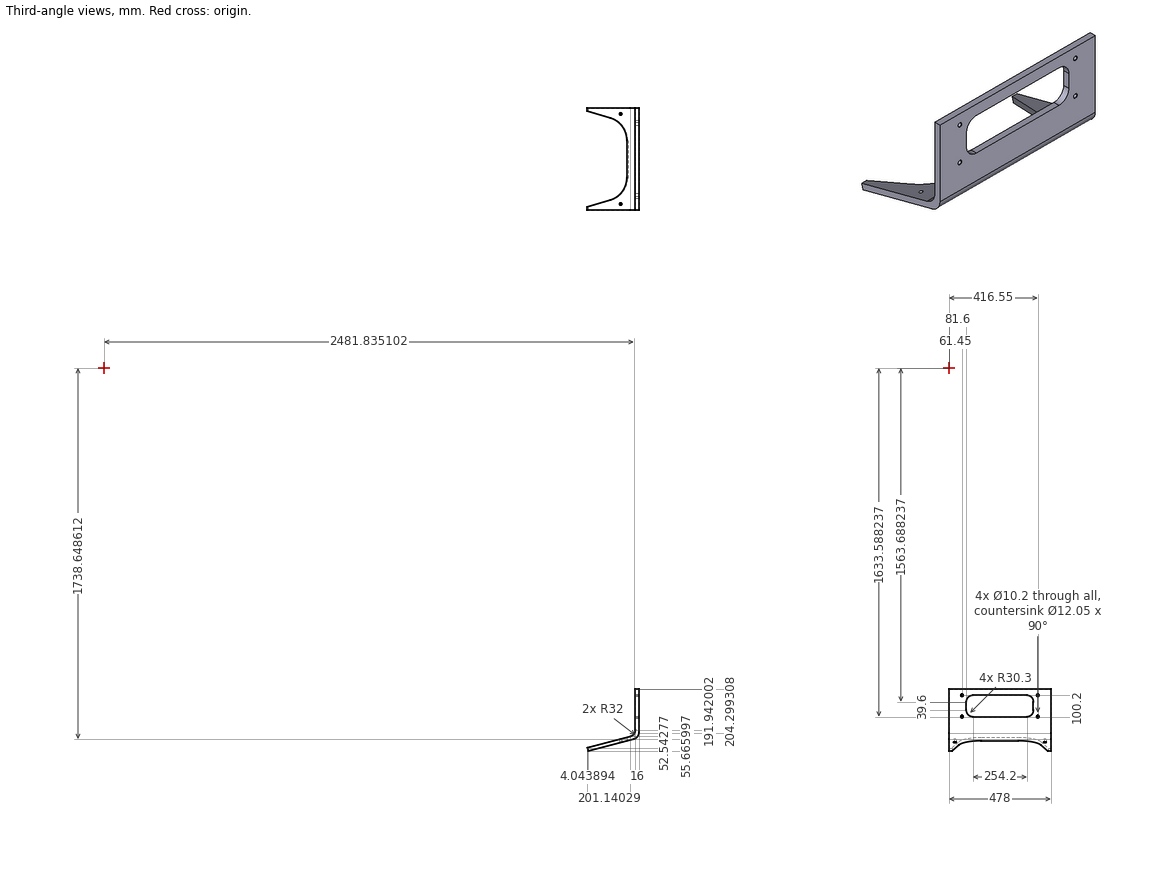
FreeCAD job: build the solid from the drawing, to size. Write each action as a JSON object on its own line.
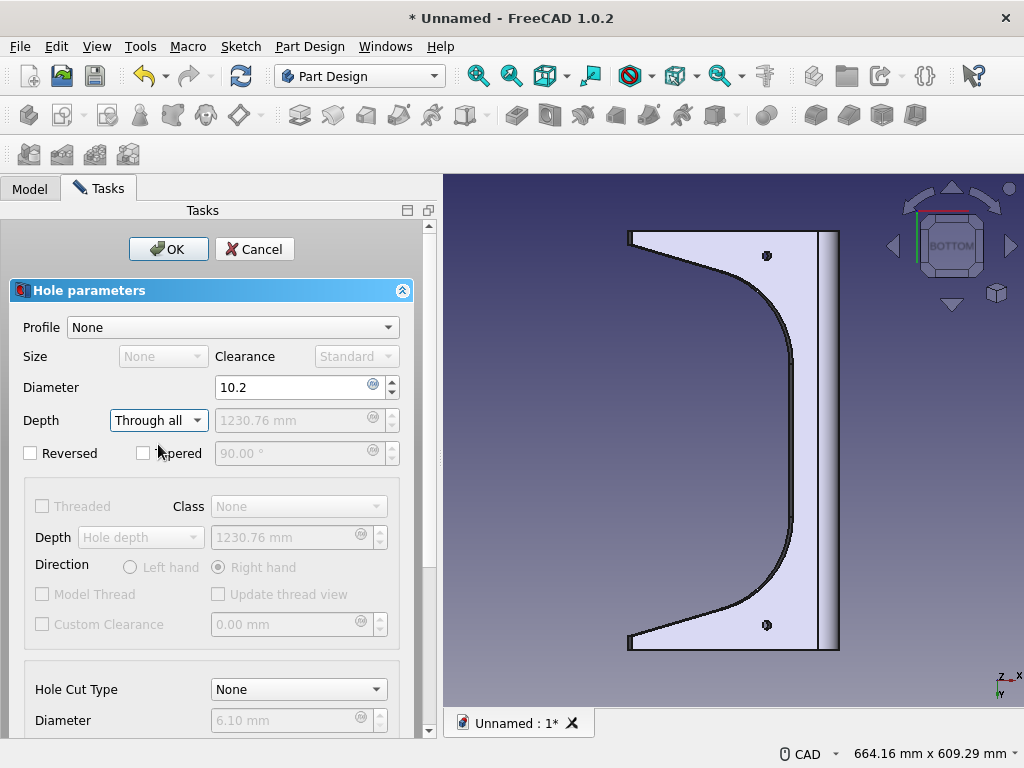
{"action": "left_click", "coordinate": [300, 690]}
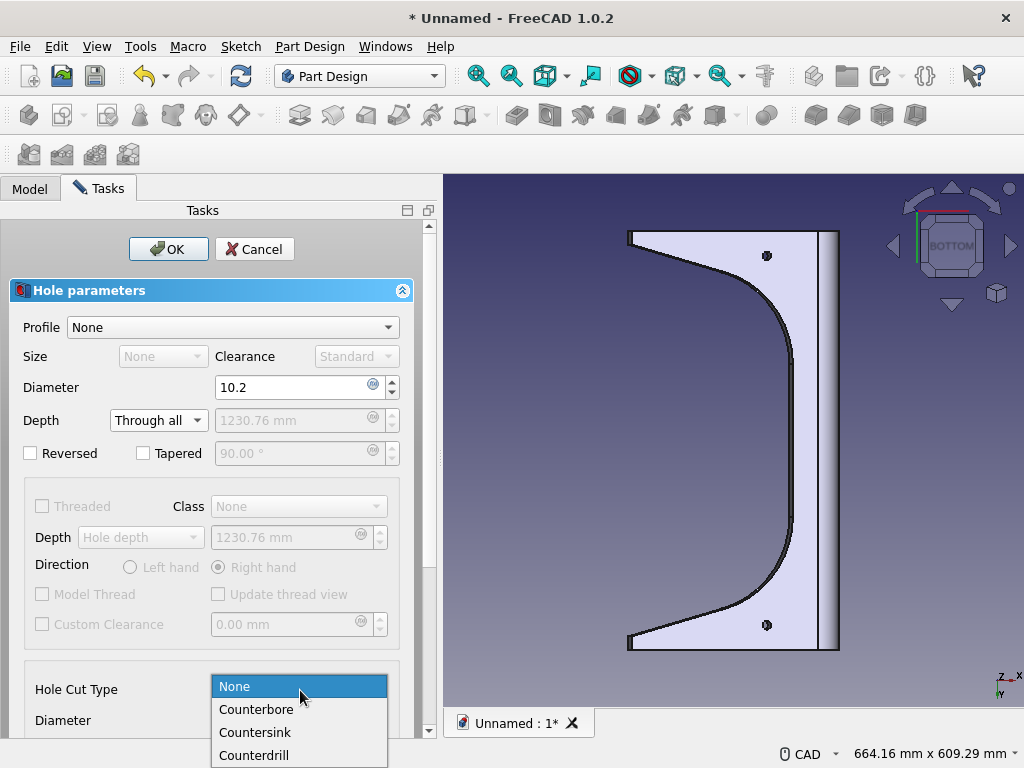
{"action": "left_click", "coordinate": [298, 732]}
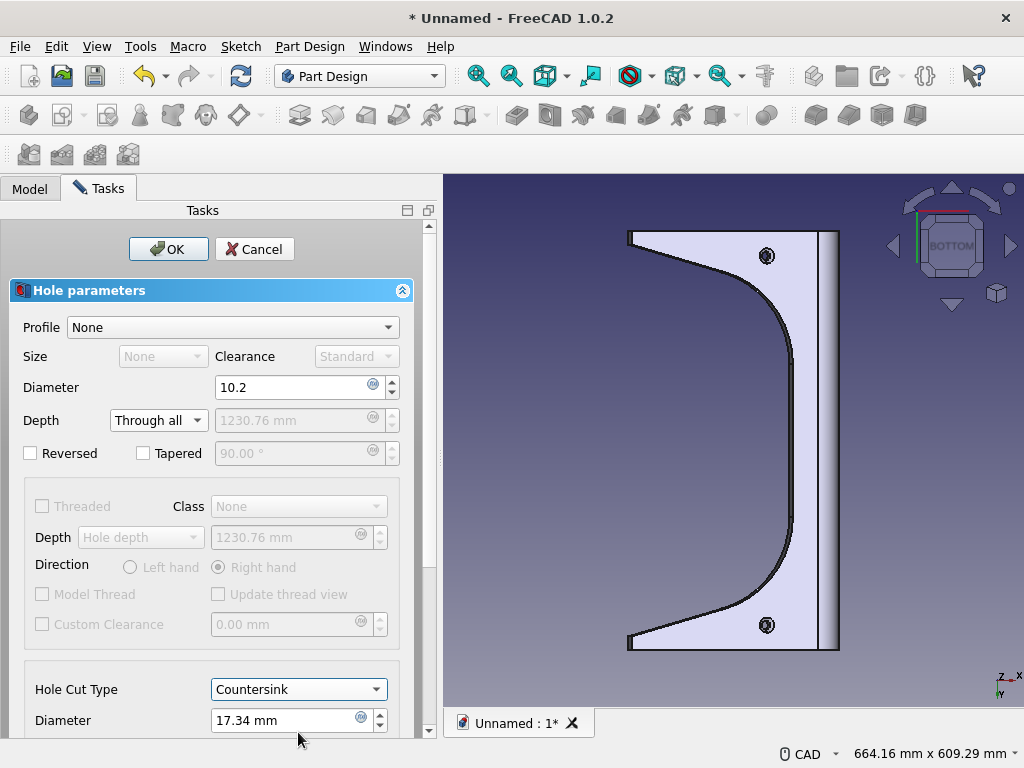
{"action": "triple_click", "coordinate": [292, 720]}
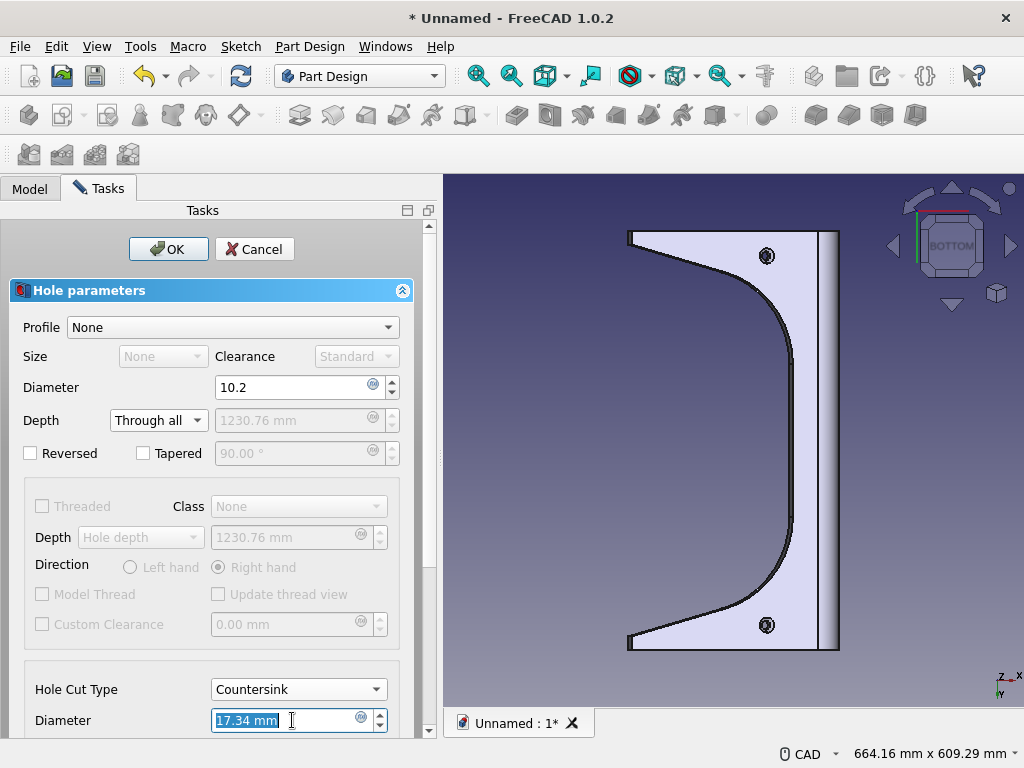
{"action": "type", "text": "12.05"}
{"action": "key", "text": "Tab"}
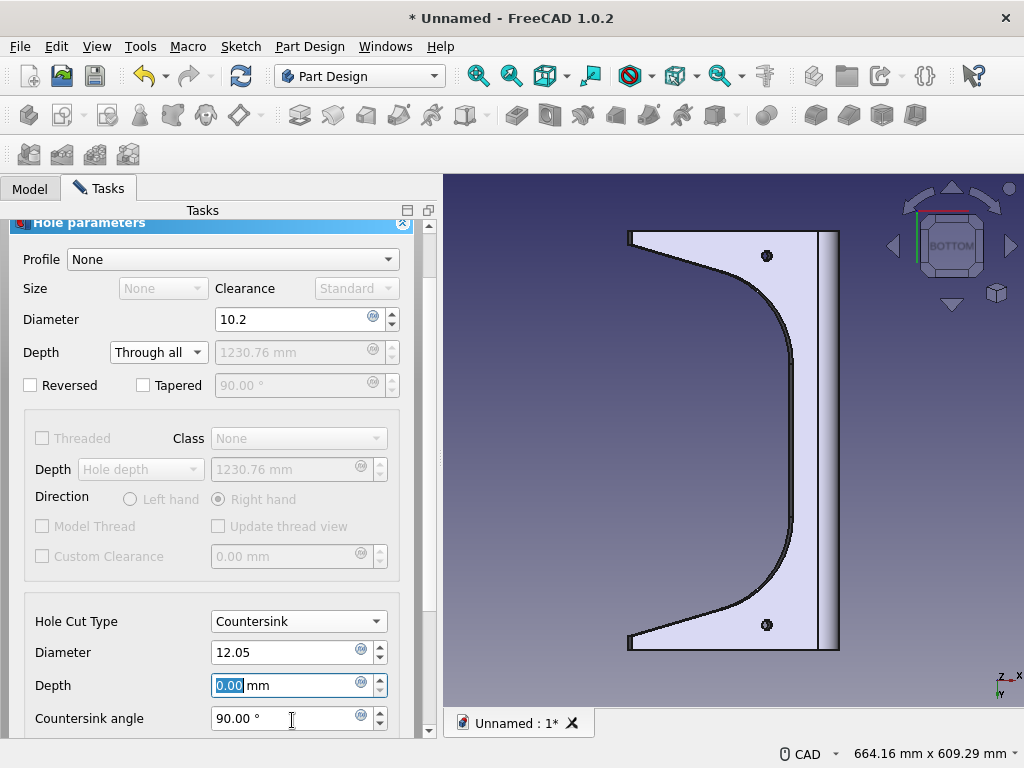
{"action": "scroll", "coordinate": [429, 479], "scroll_direction": "up", "scroll_amount": 2}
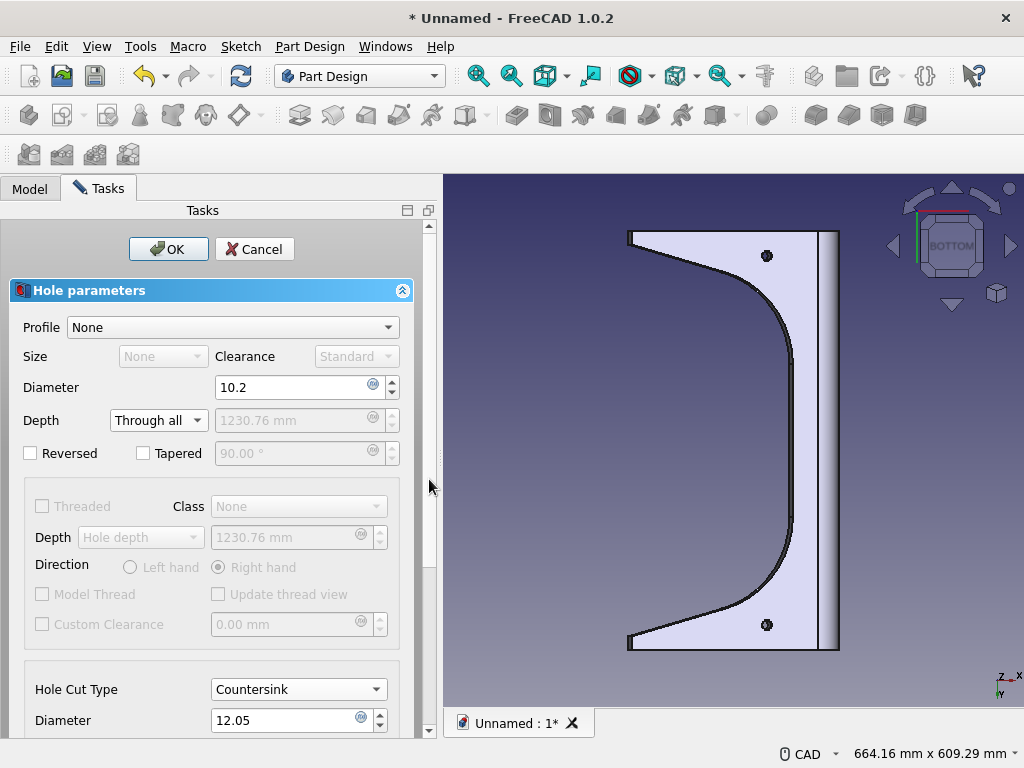
{"action": "left_click", "coordinate": [169, 249]}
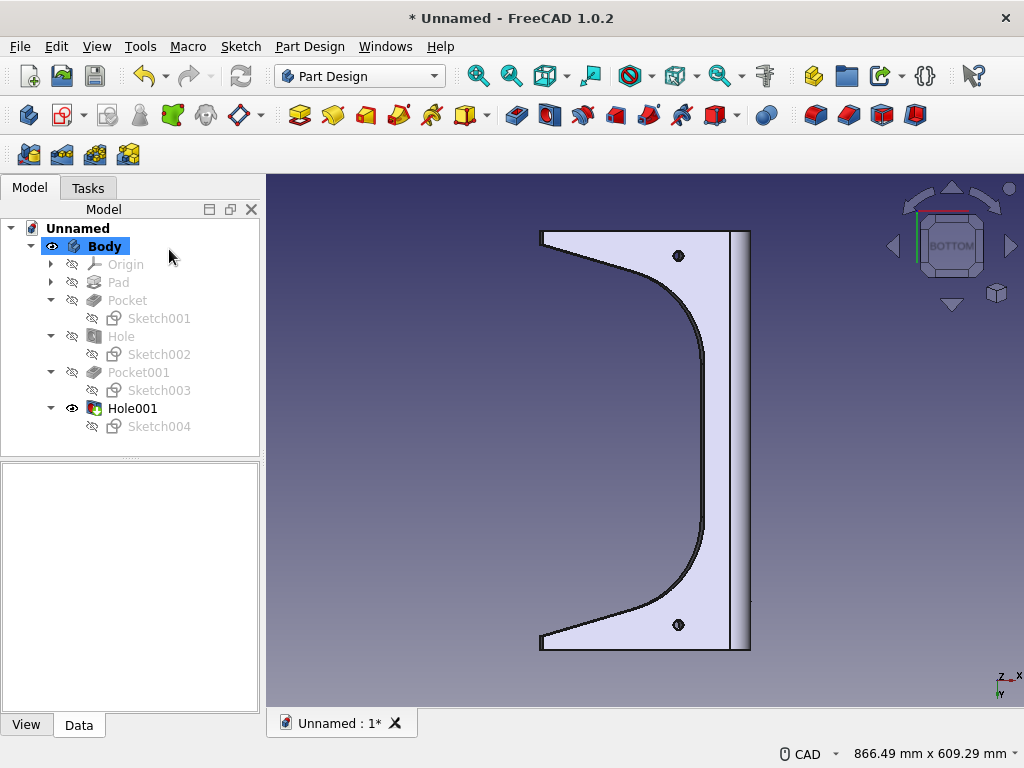
{"action": "key", "text": "0"}